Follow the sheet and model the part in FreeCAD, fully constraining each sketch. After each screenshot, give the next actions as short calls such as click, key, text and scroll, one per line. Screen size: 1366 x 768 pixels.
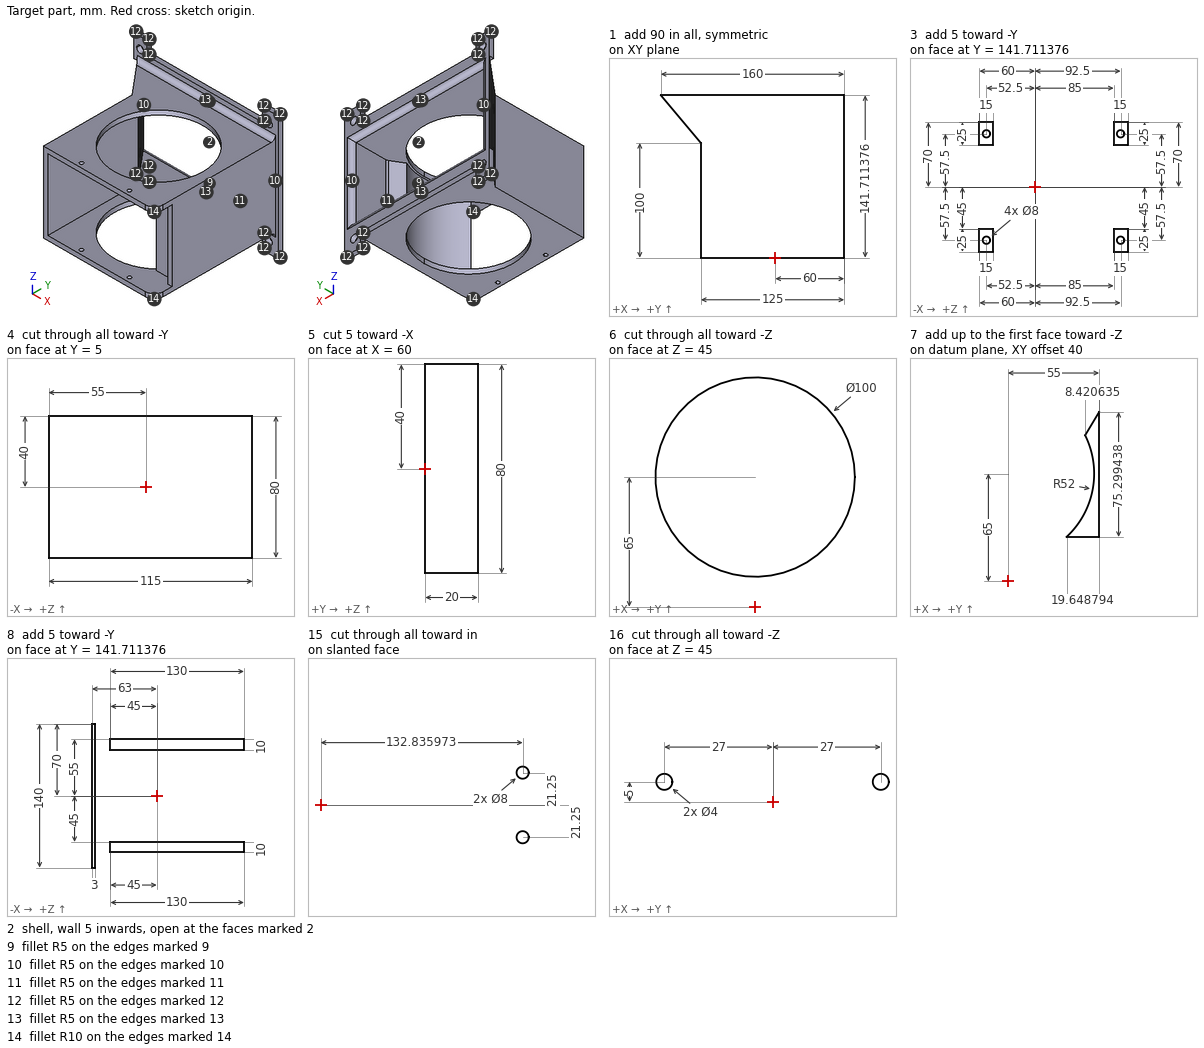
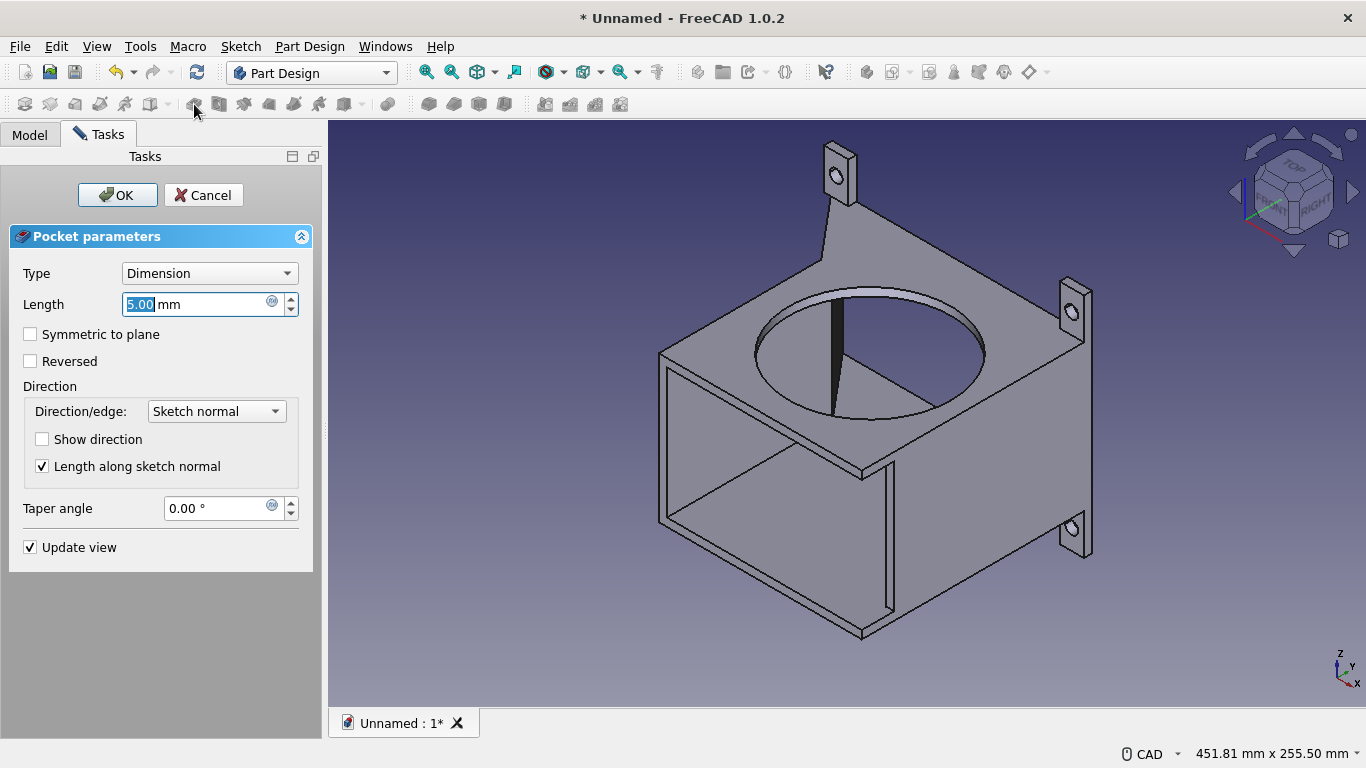
click(210, 274)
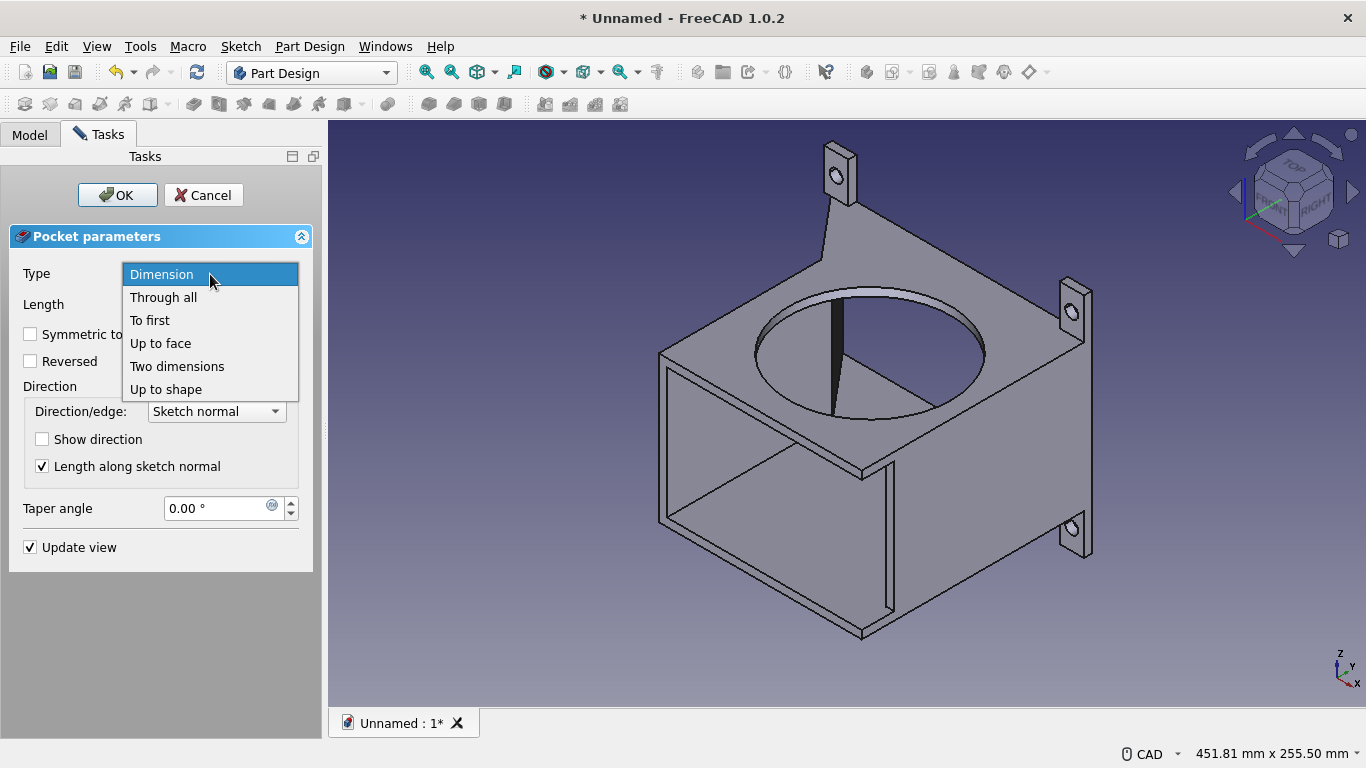
click(208, 298)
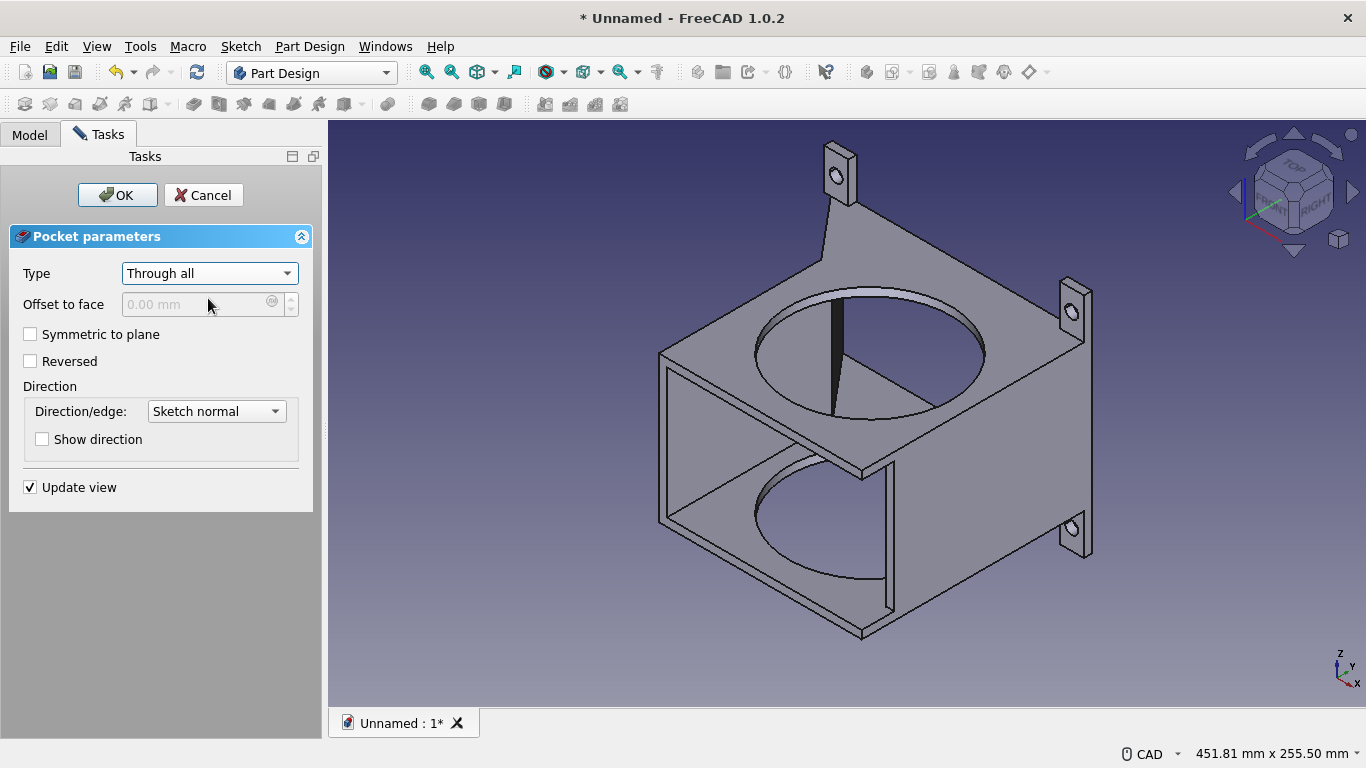
click(118, 195)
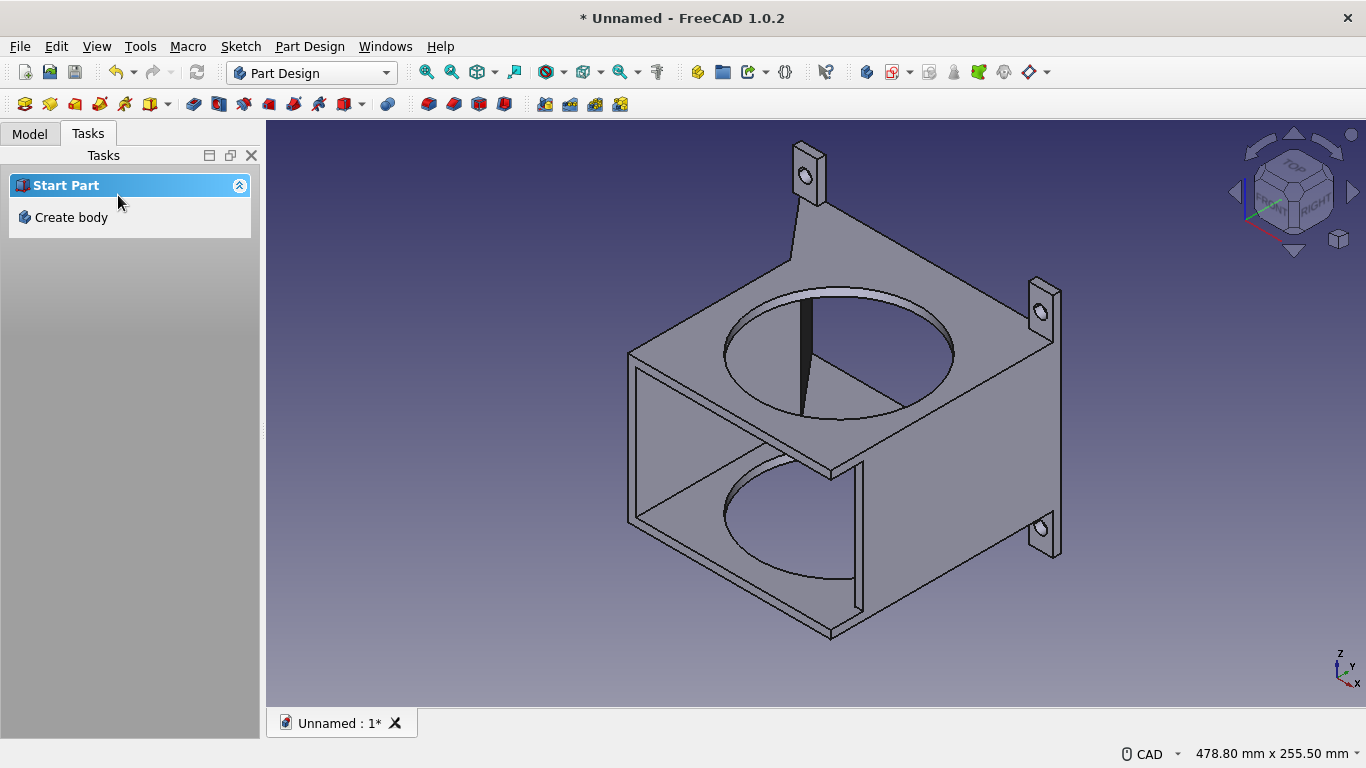
click(30, 134)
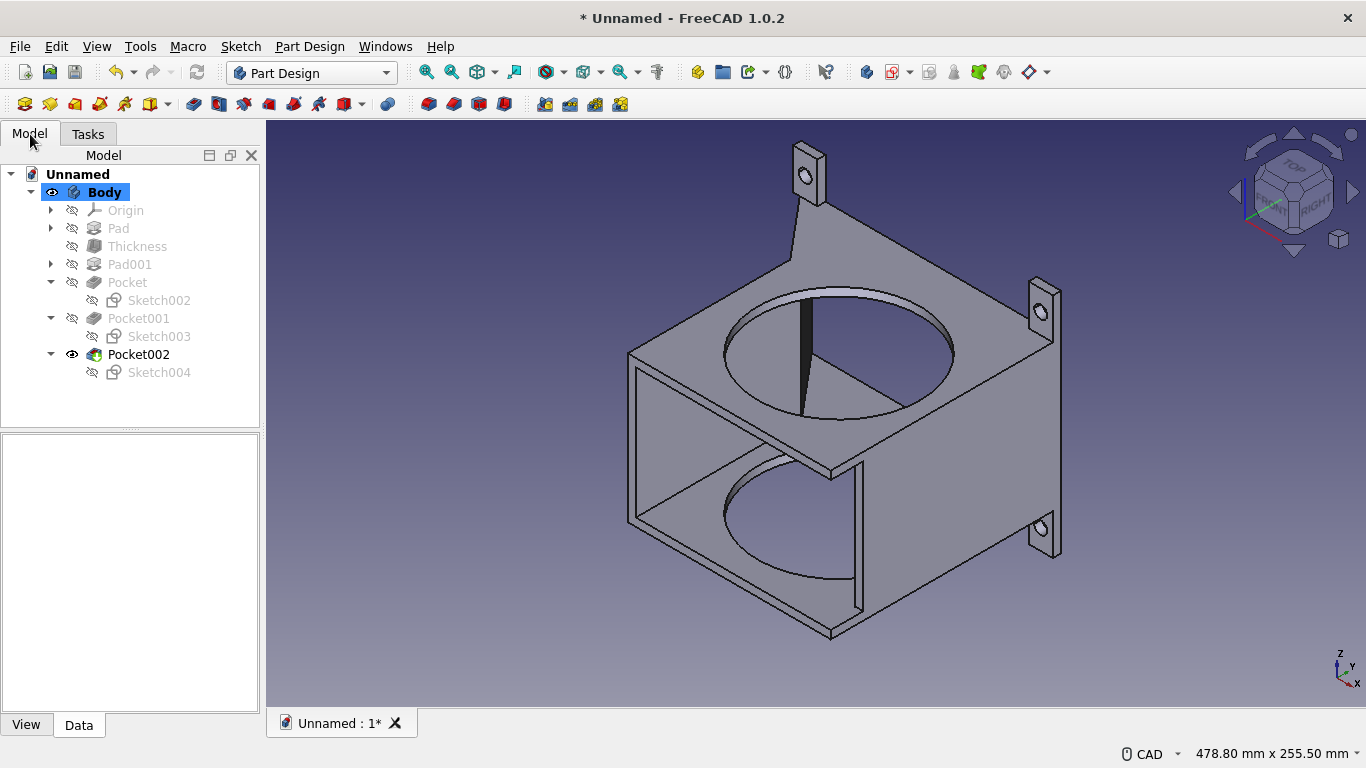
click(51, 210)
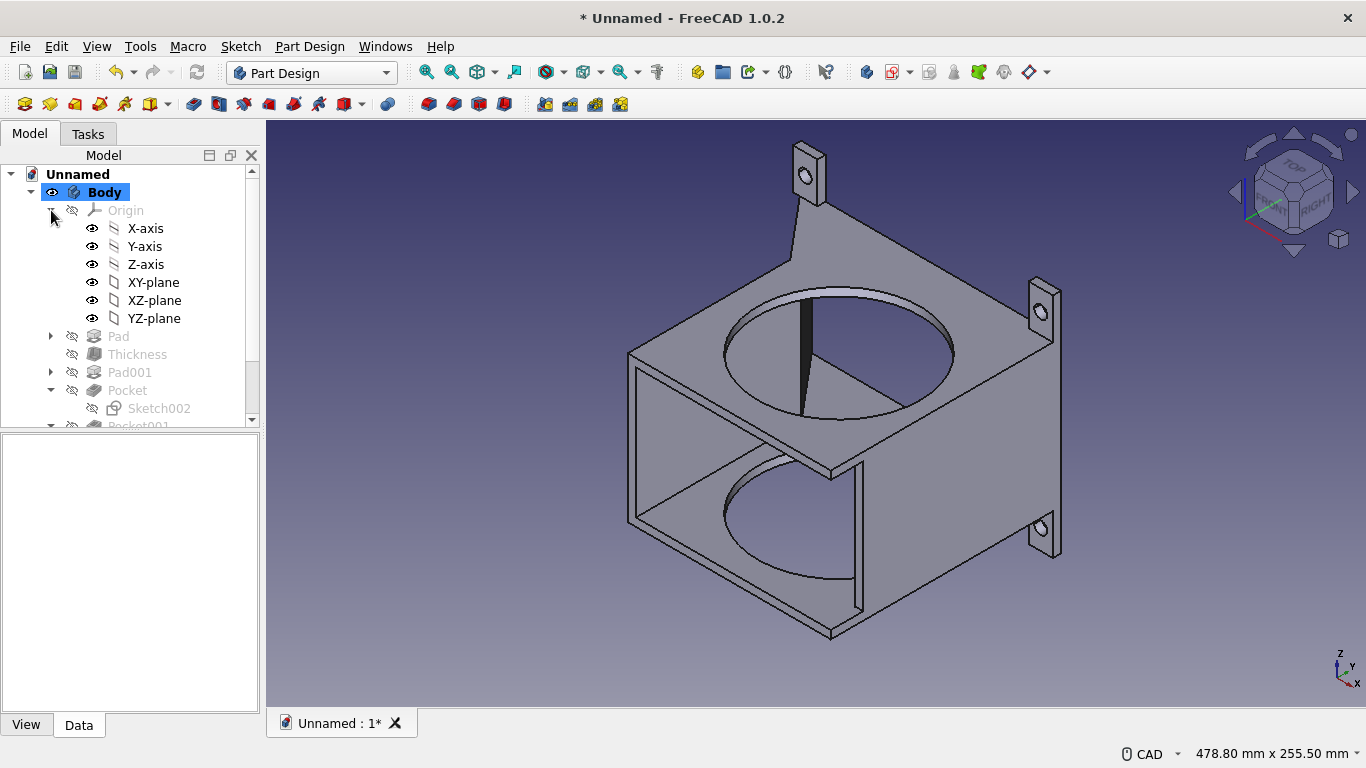
click(137, 282)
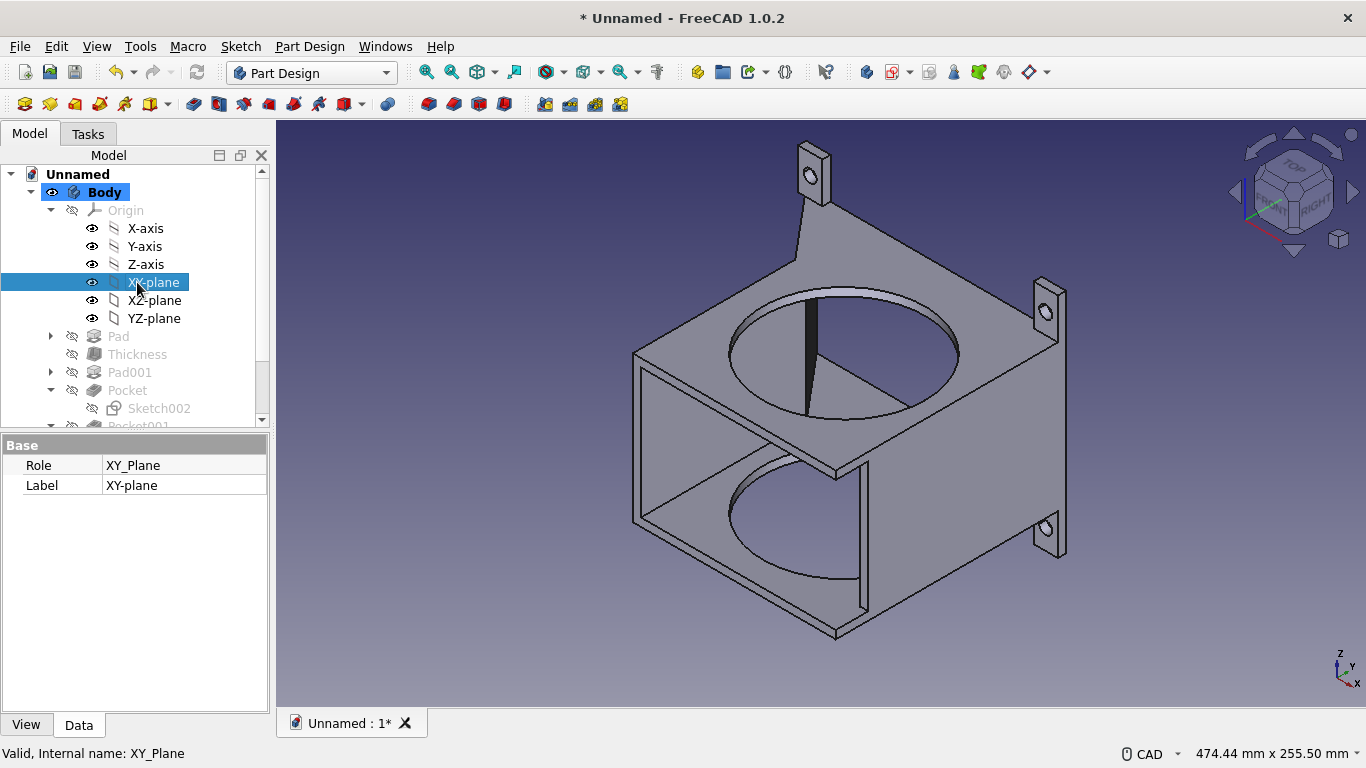
click(1028, 72)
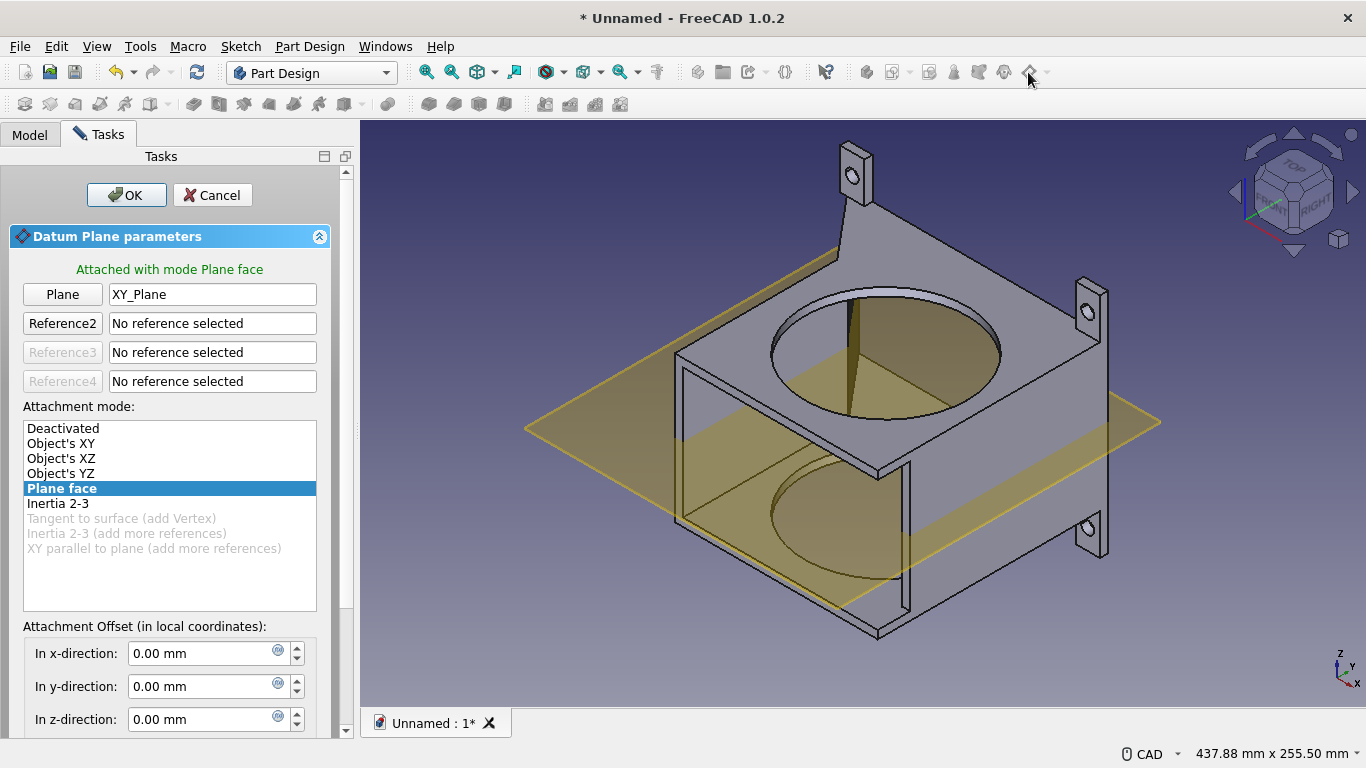
triple_click(210, 720)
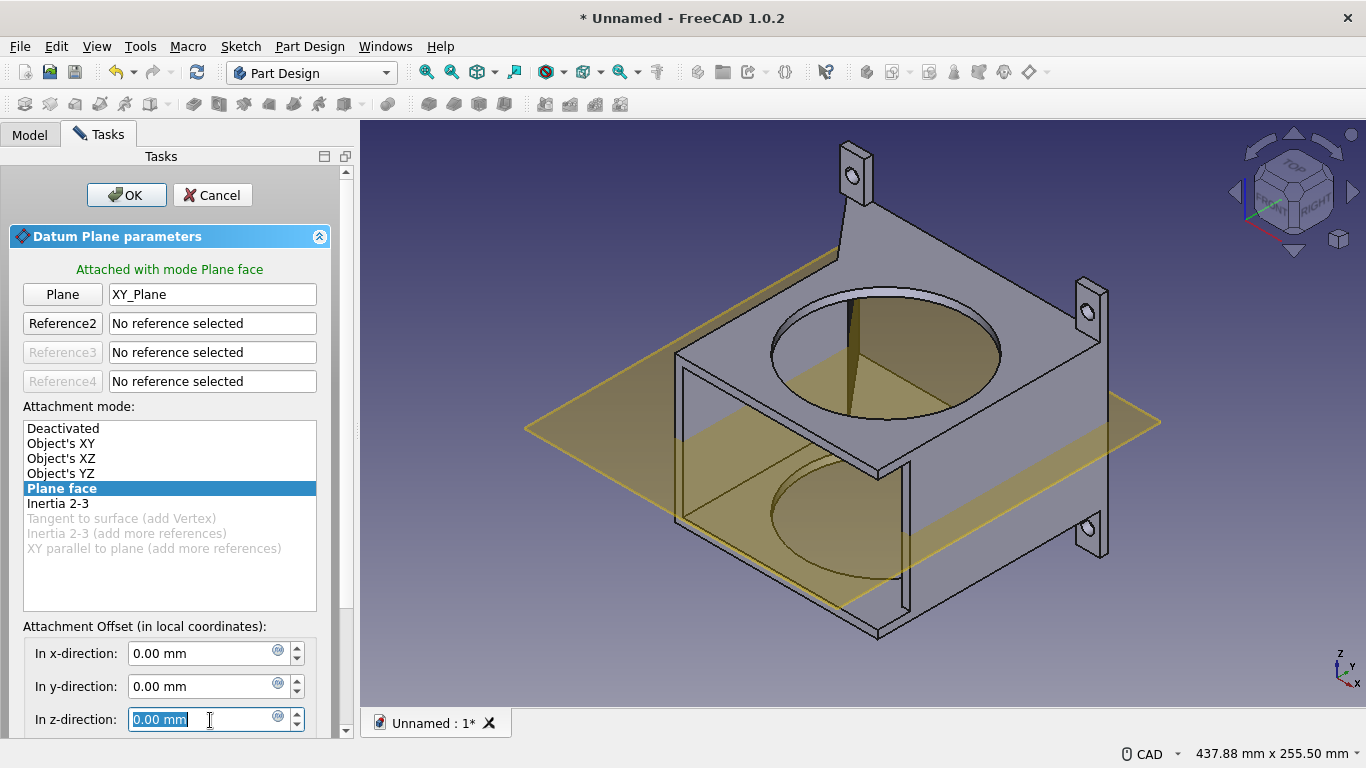
text(40)
key(Tab)